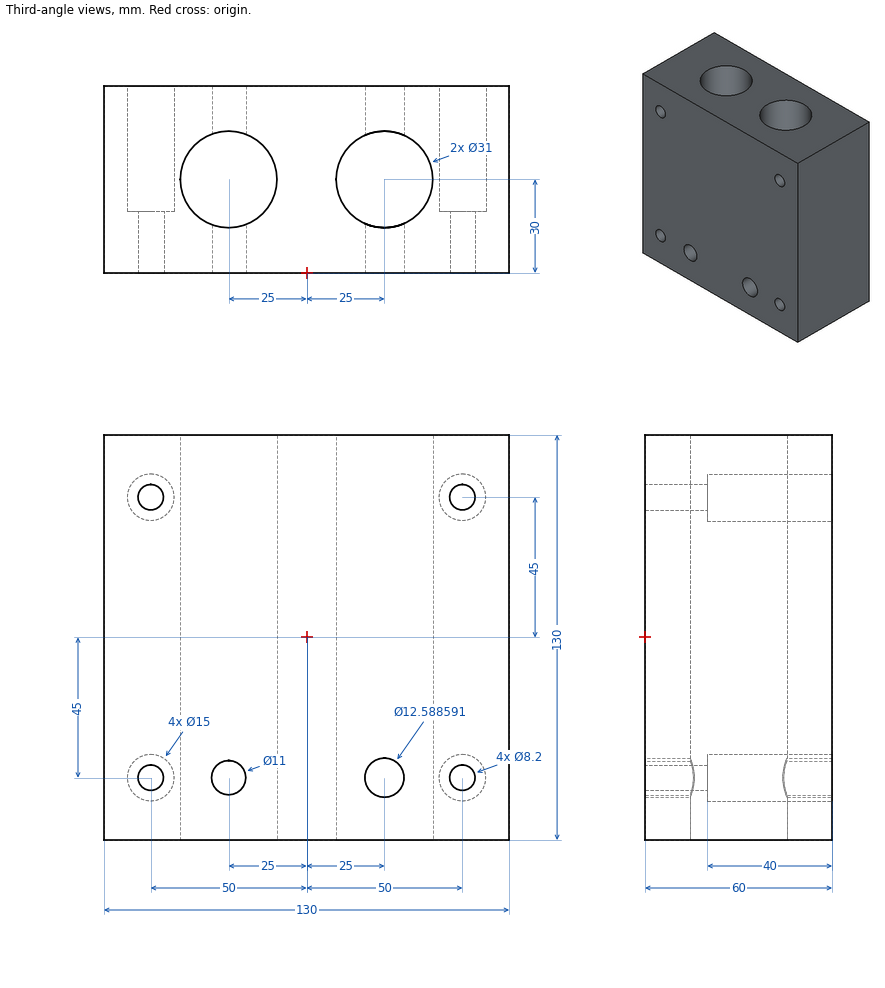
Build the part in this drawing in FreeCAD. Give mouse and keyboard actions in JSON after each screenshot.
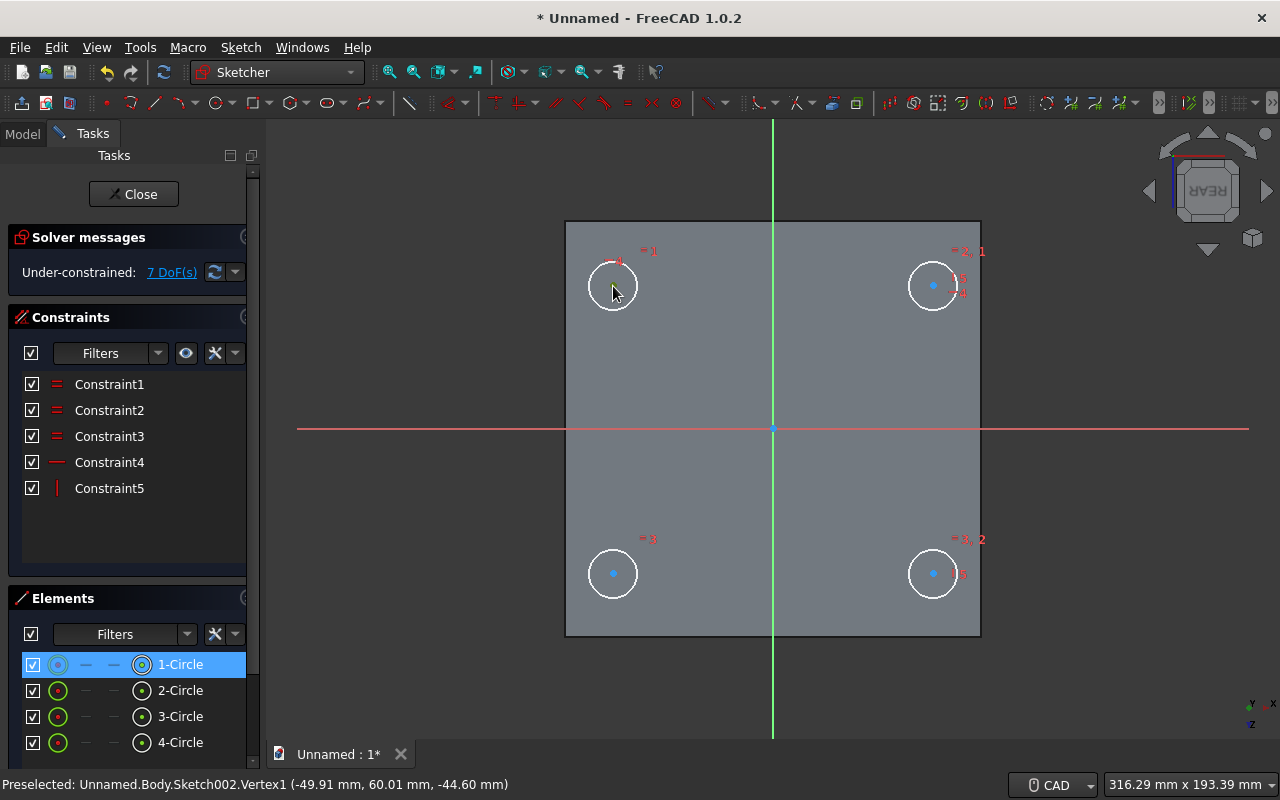
{"action": "left_click", "coordinate": [613, 574]}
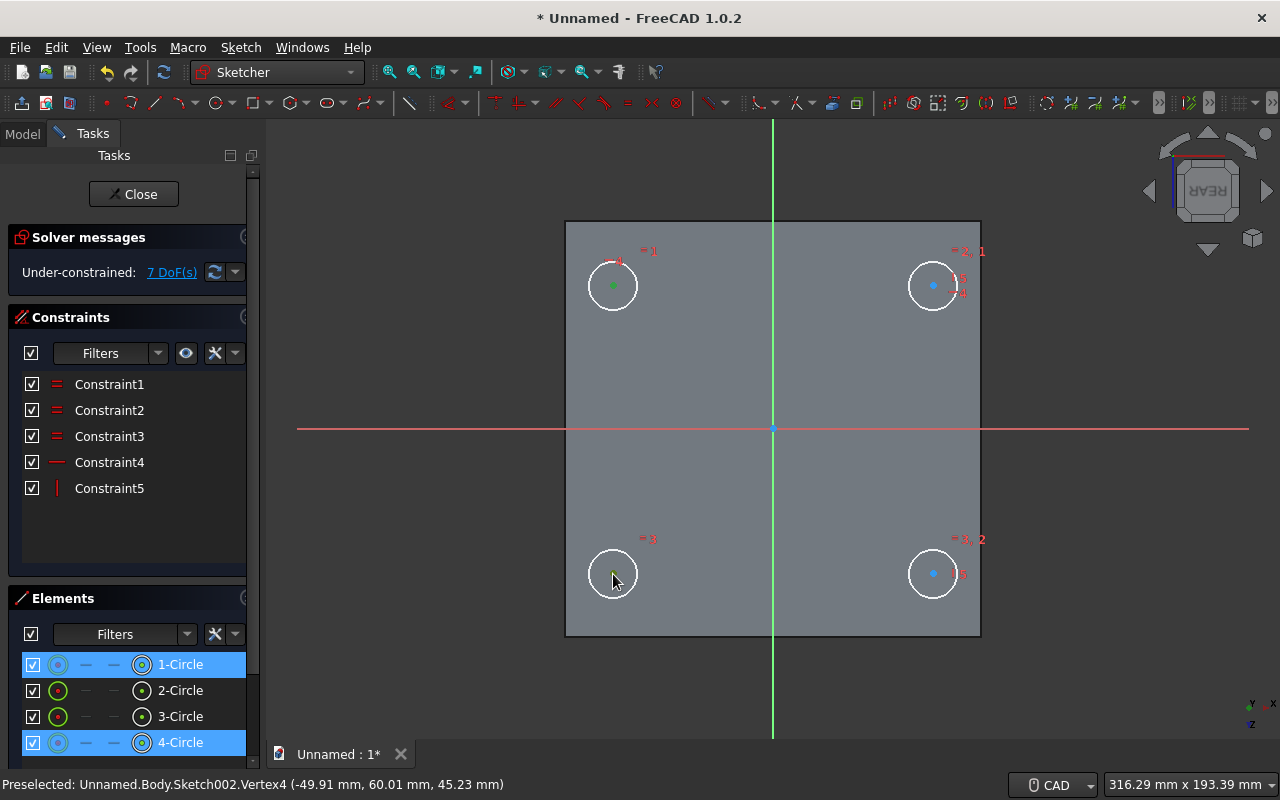
{"action": "key", "text": "v"}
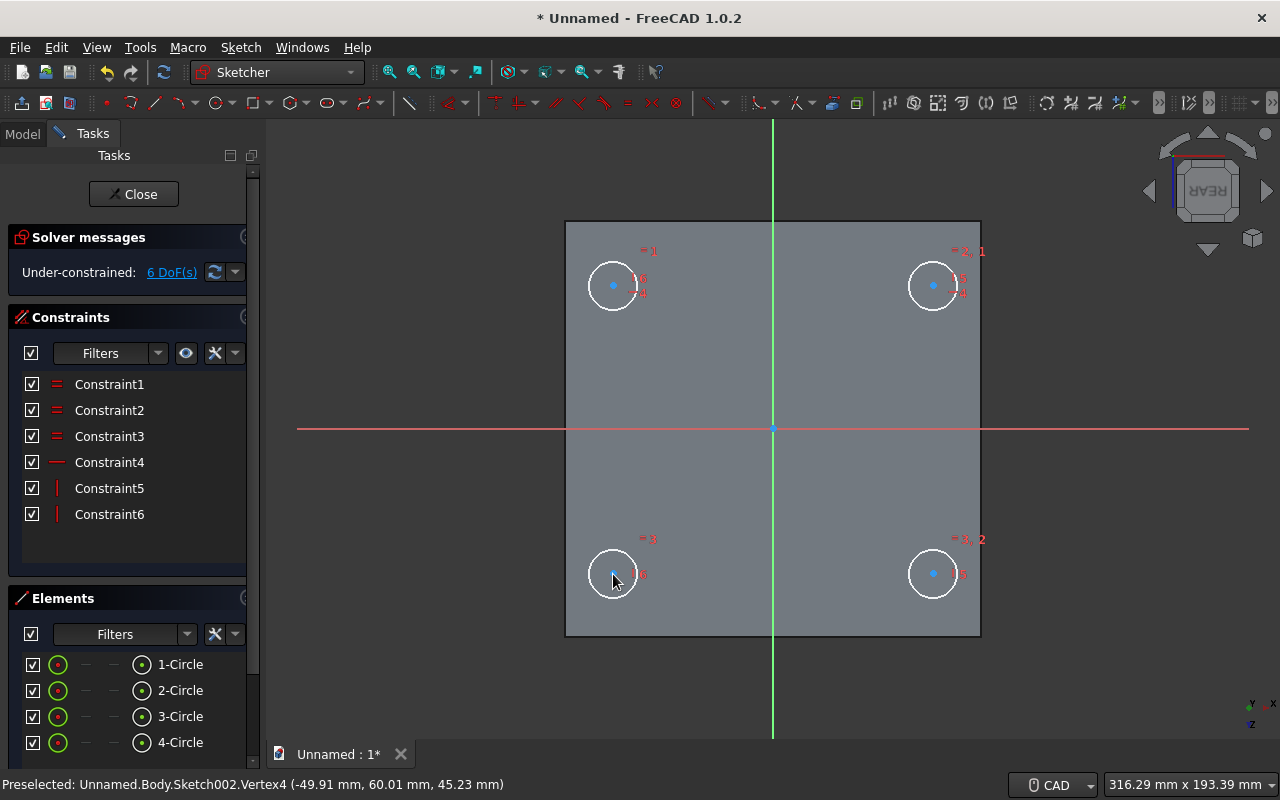
{"action": "left_click", "coordinate": [933, 574]}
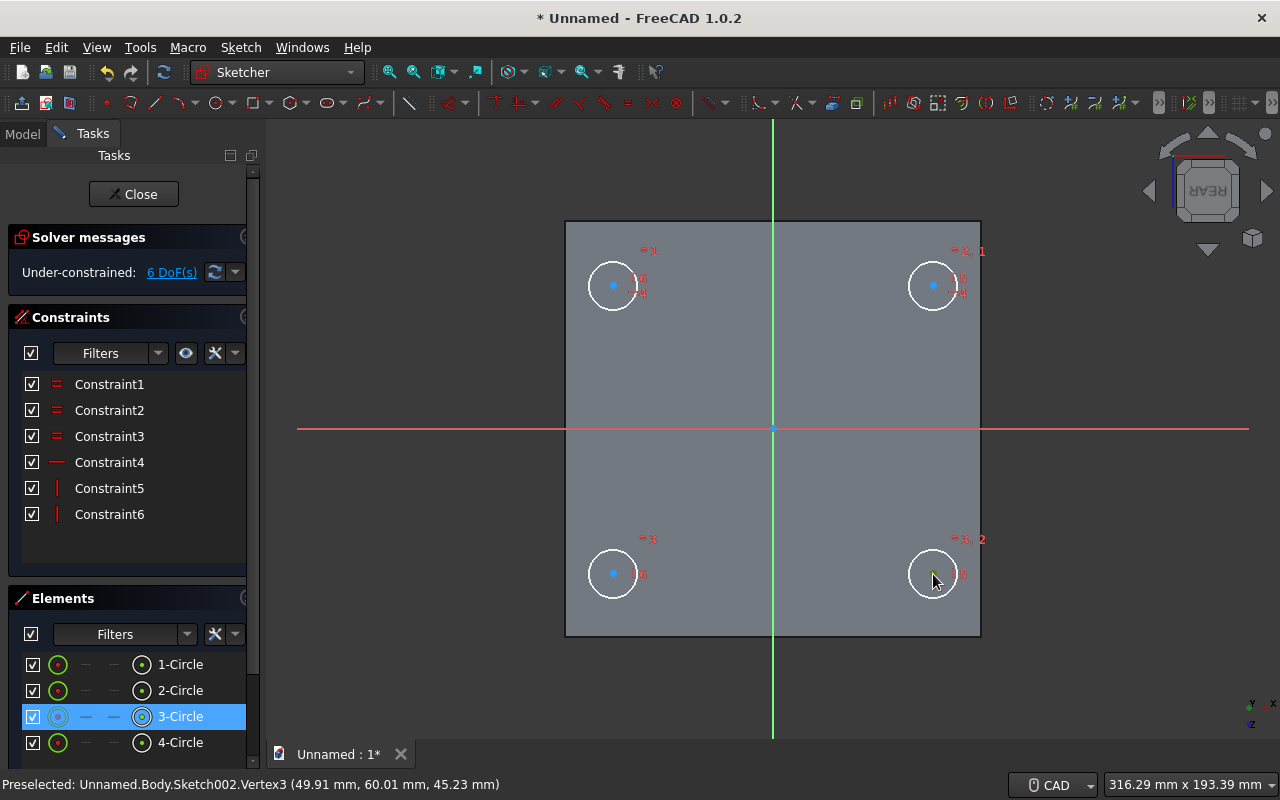
{"action": "left_click", "coordinate": [613, 574]}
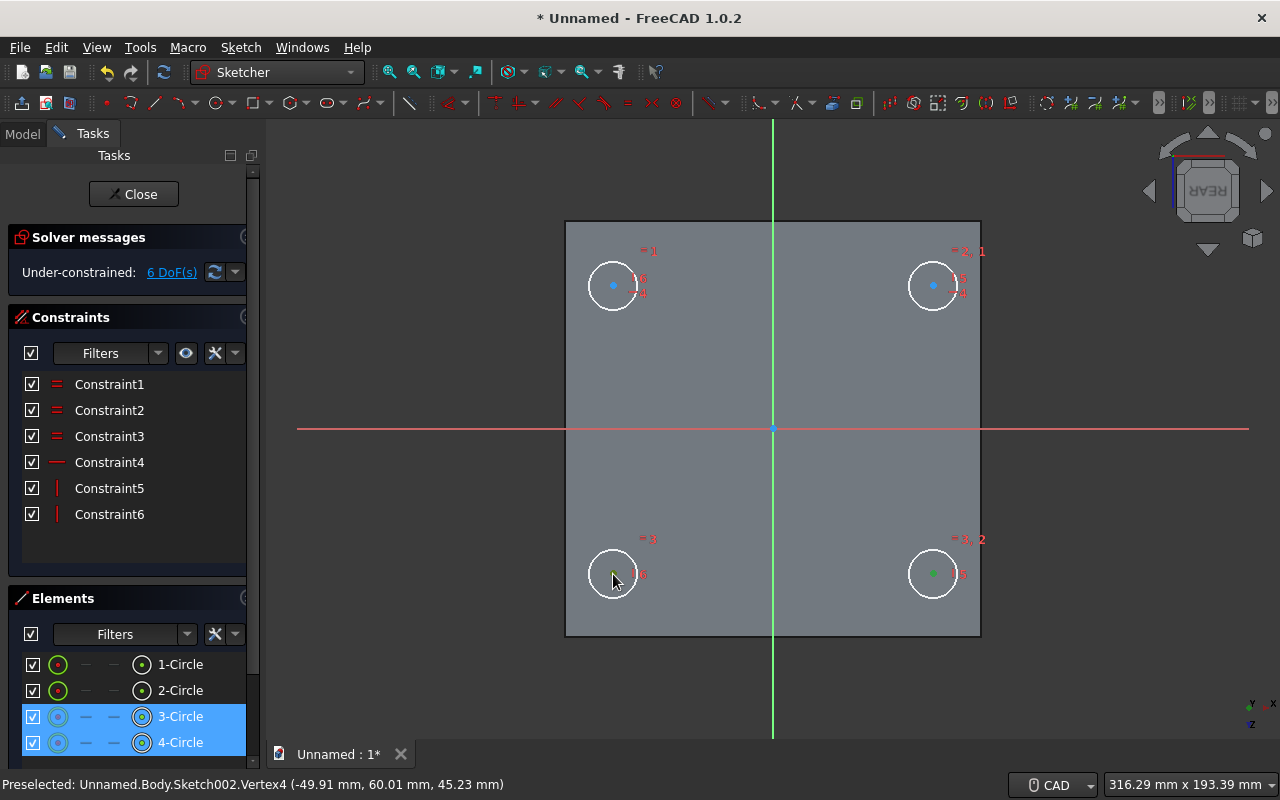
{"action": "key", "text": "h"}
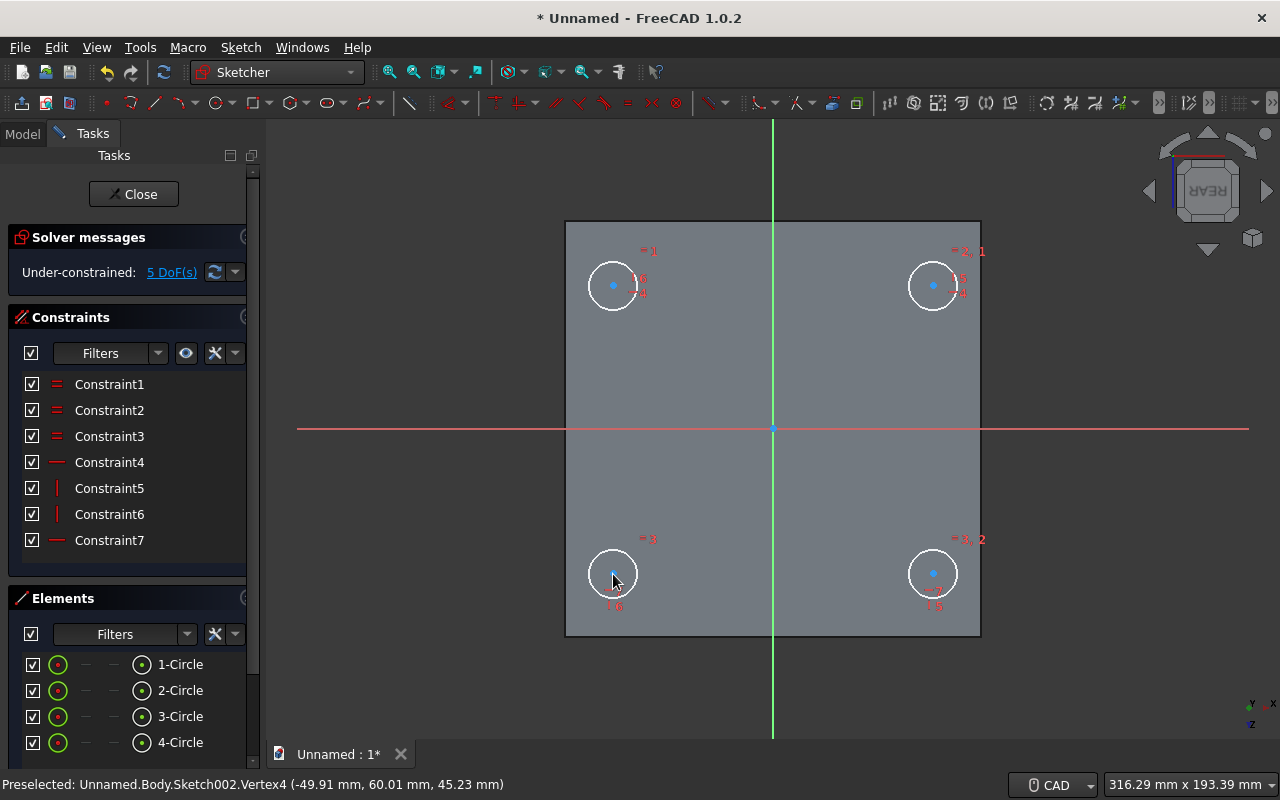
{"action": "left_click", "coordinate": [630, 269]}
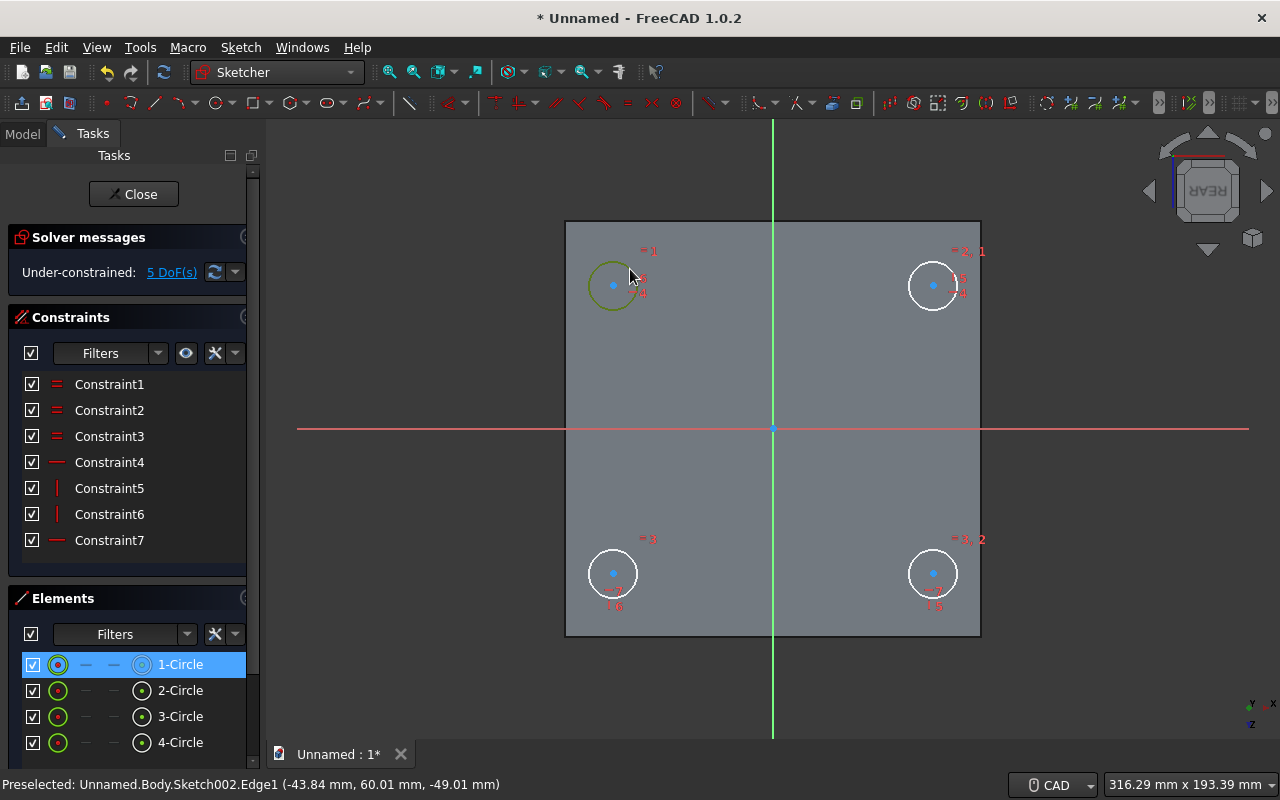
{"action": "key", "text": "k o"}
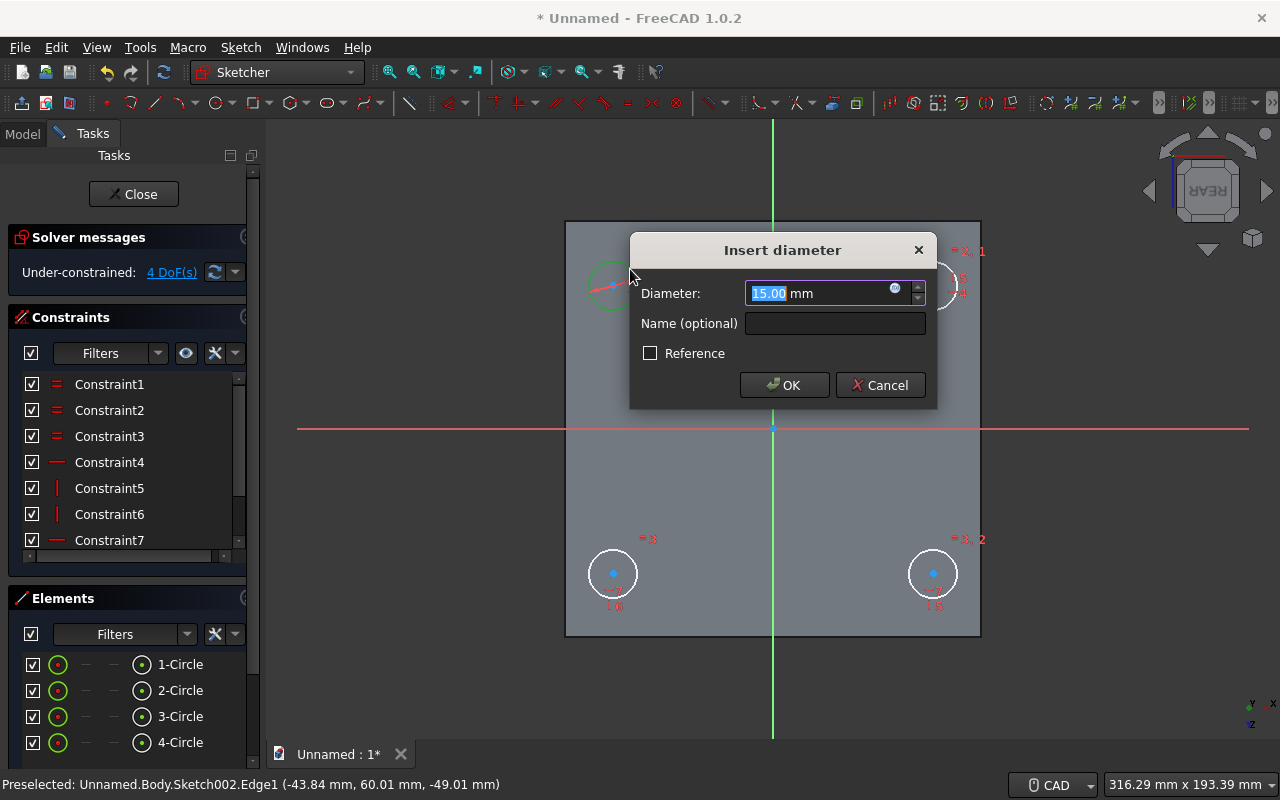
{"action": "type", "text": "15"}
{"action": "key", "text": "Return"}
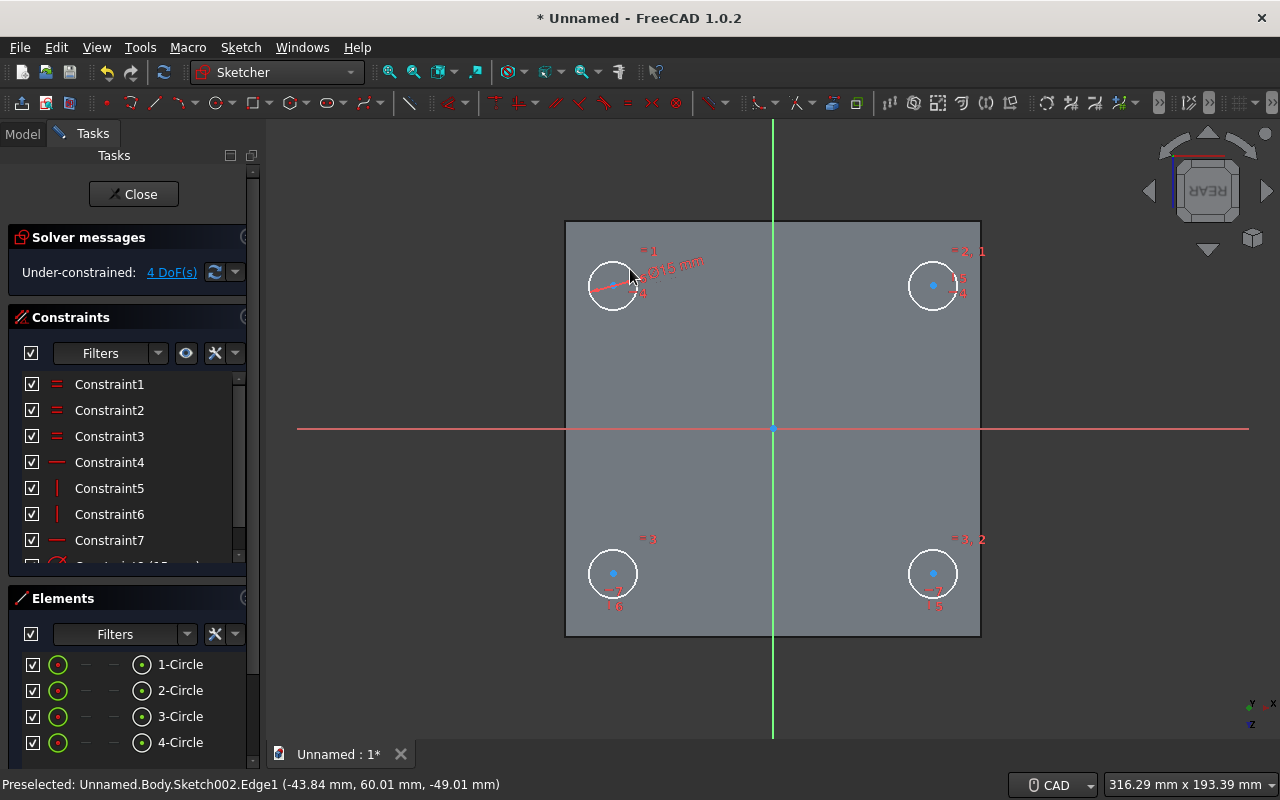
{"action": "left_click", "coordinate": [613, 286]}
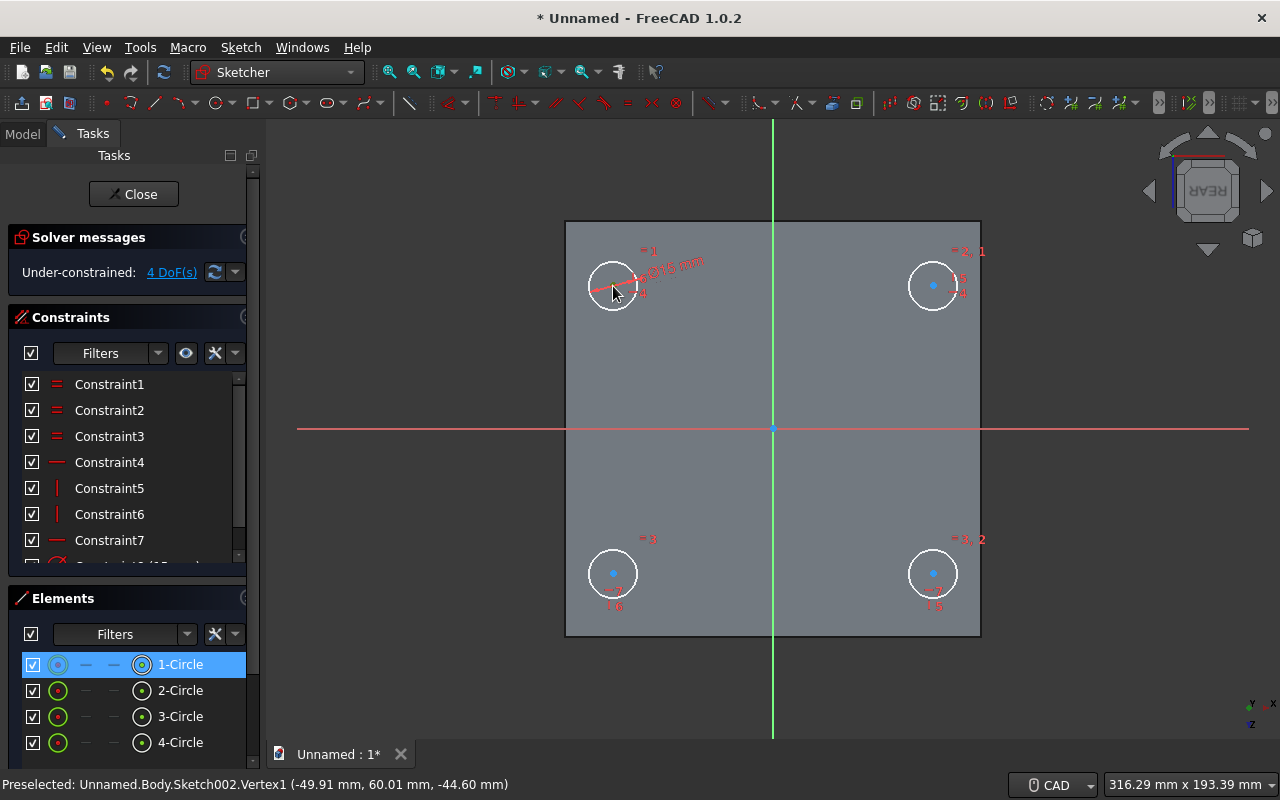
{"action": "left_click", "coordinate": [468, 104]}